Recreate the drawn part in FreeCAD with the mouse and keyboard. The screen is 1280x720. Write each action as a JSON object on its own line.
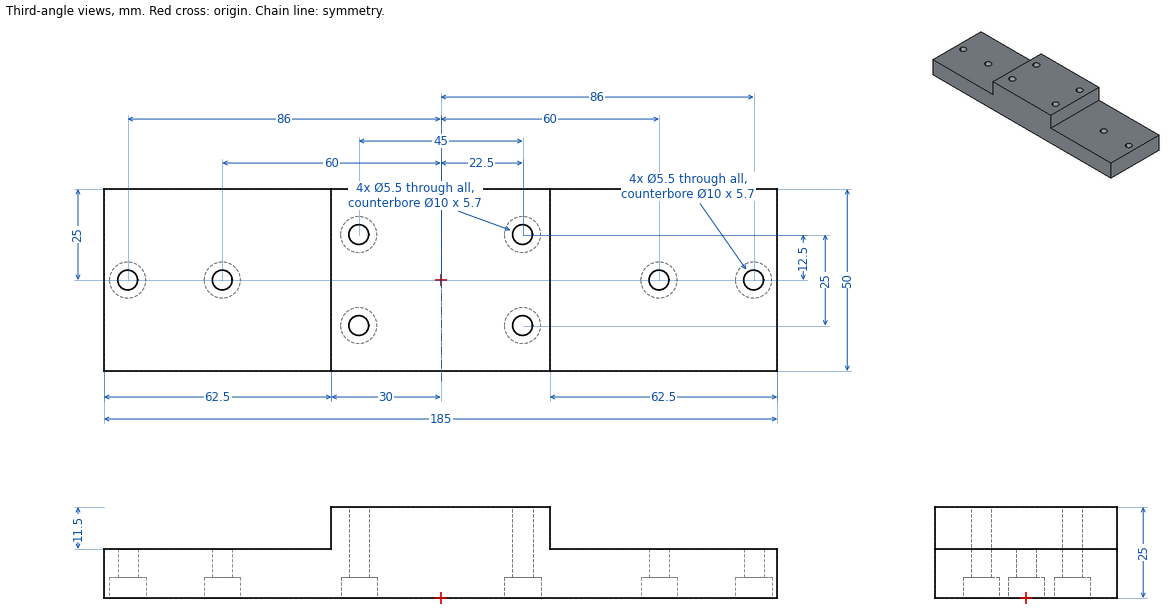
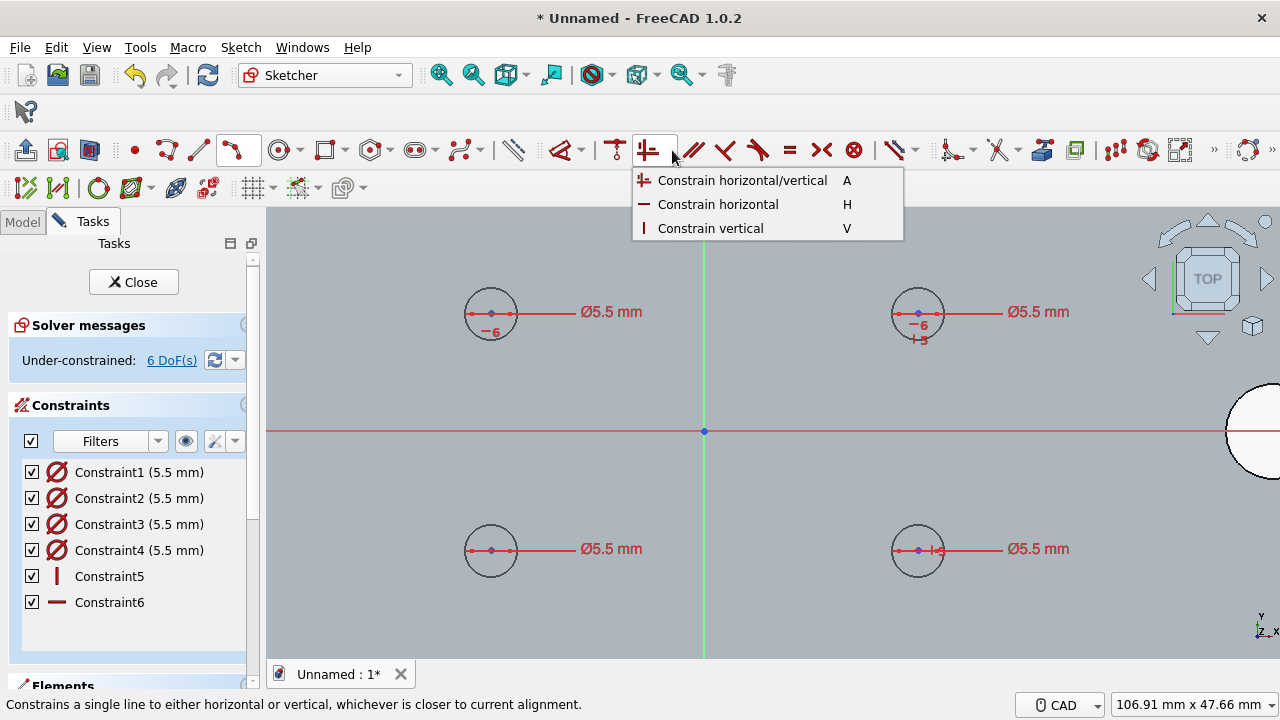
{"action": "left_click", "coordinate": [768, 228]}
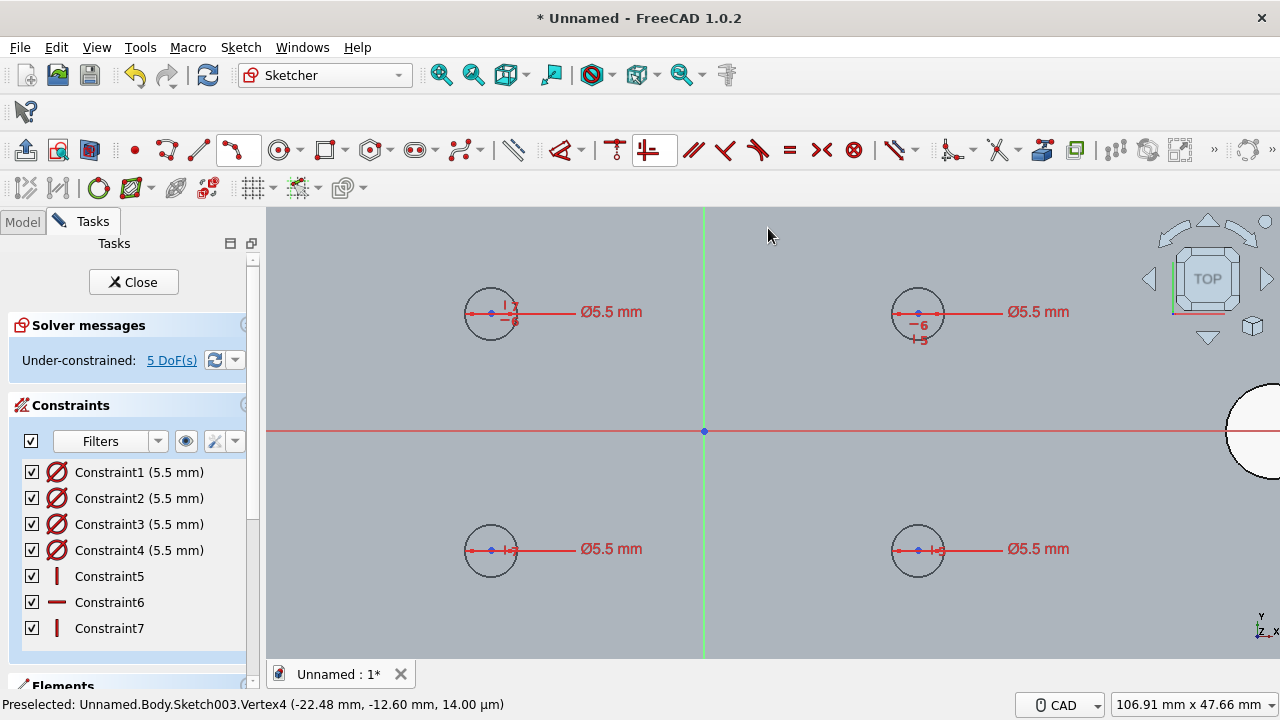
{"action": "left_click", "coordinate": [918, 551]}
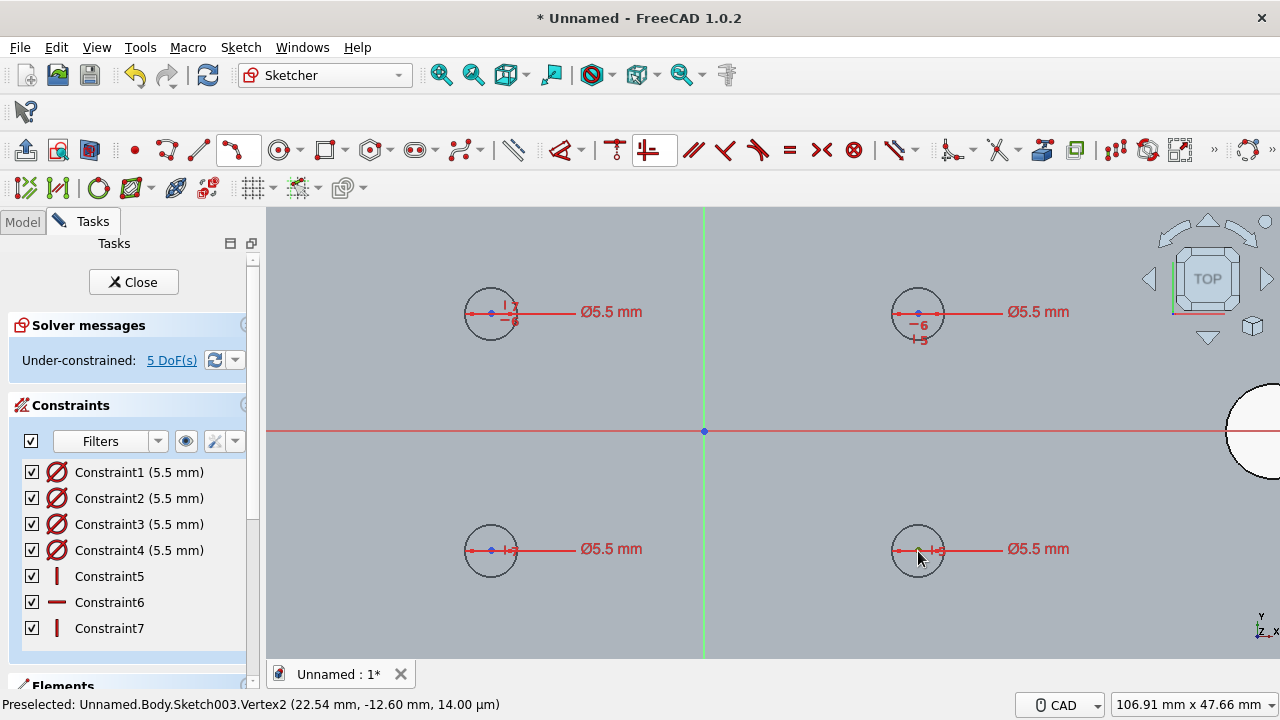
{"action": "left_click", "coordinate": [491, 551]}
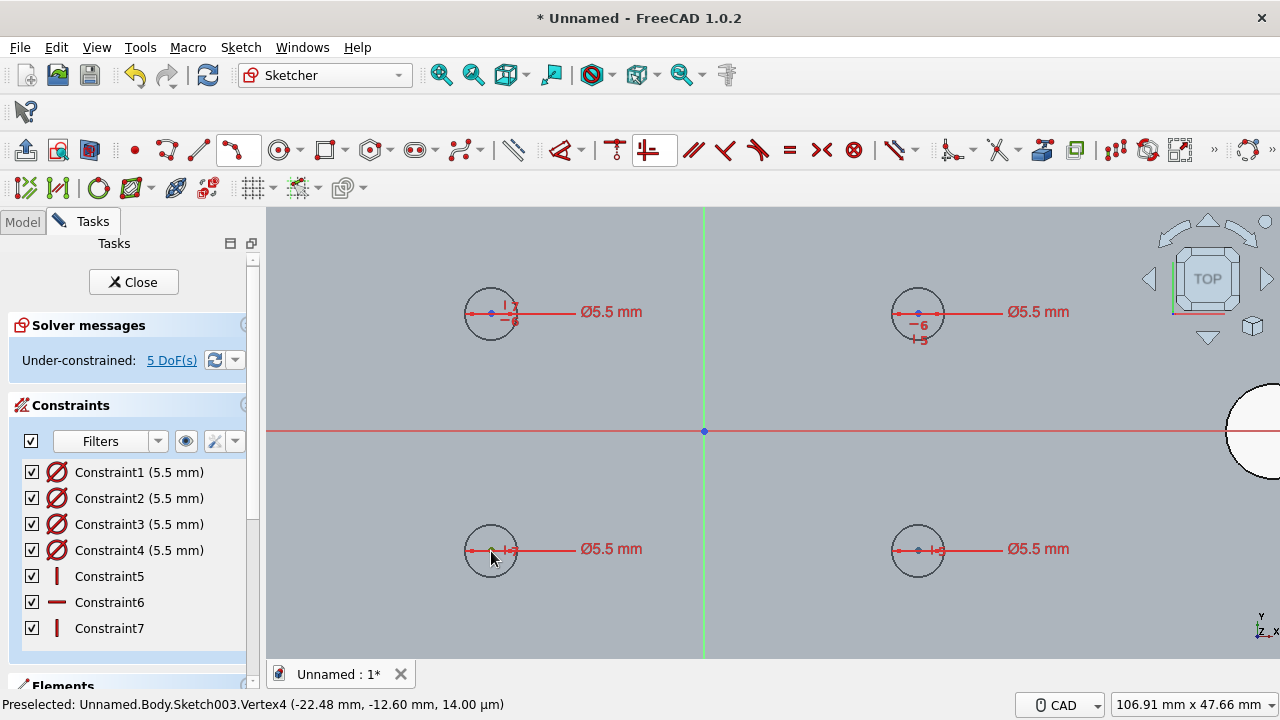
{"action": "left_click", "coordinate": [672, 150]}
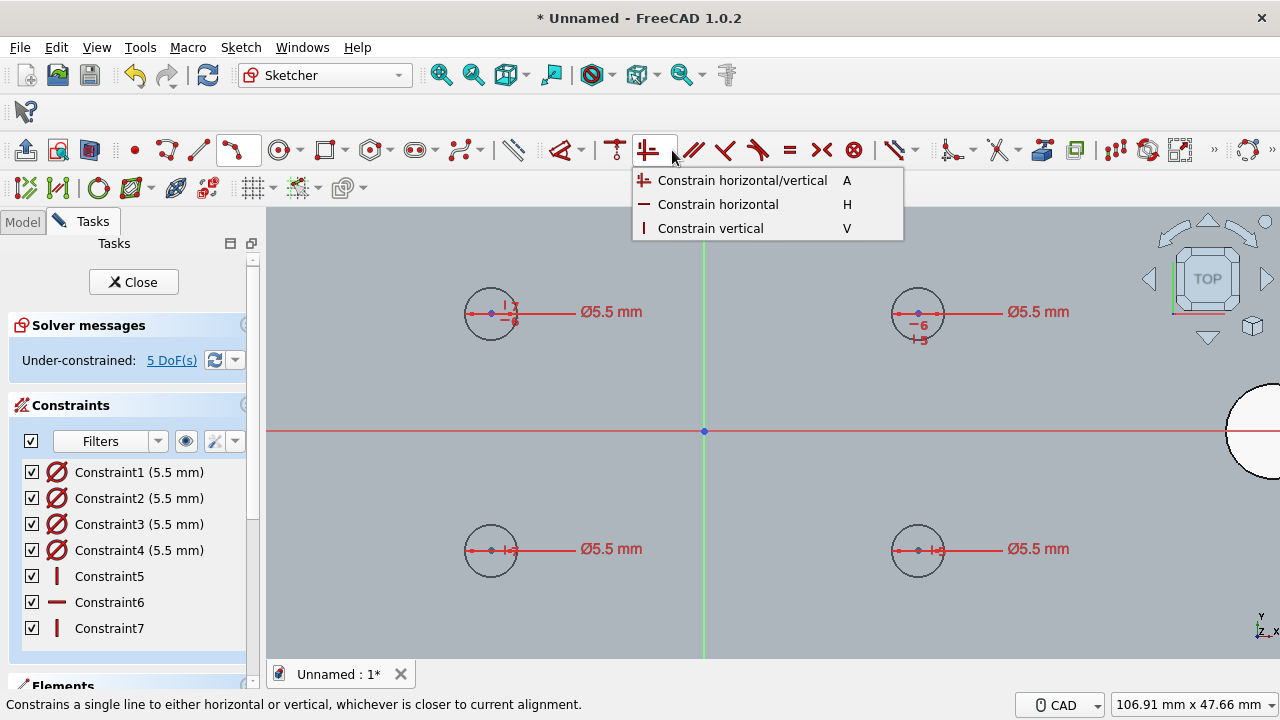
{"action": "left_click", "coordinate": [768, 204]}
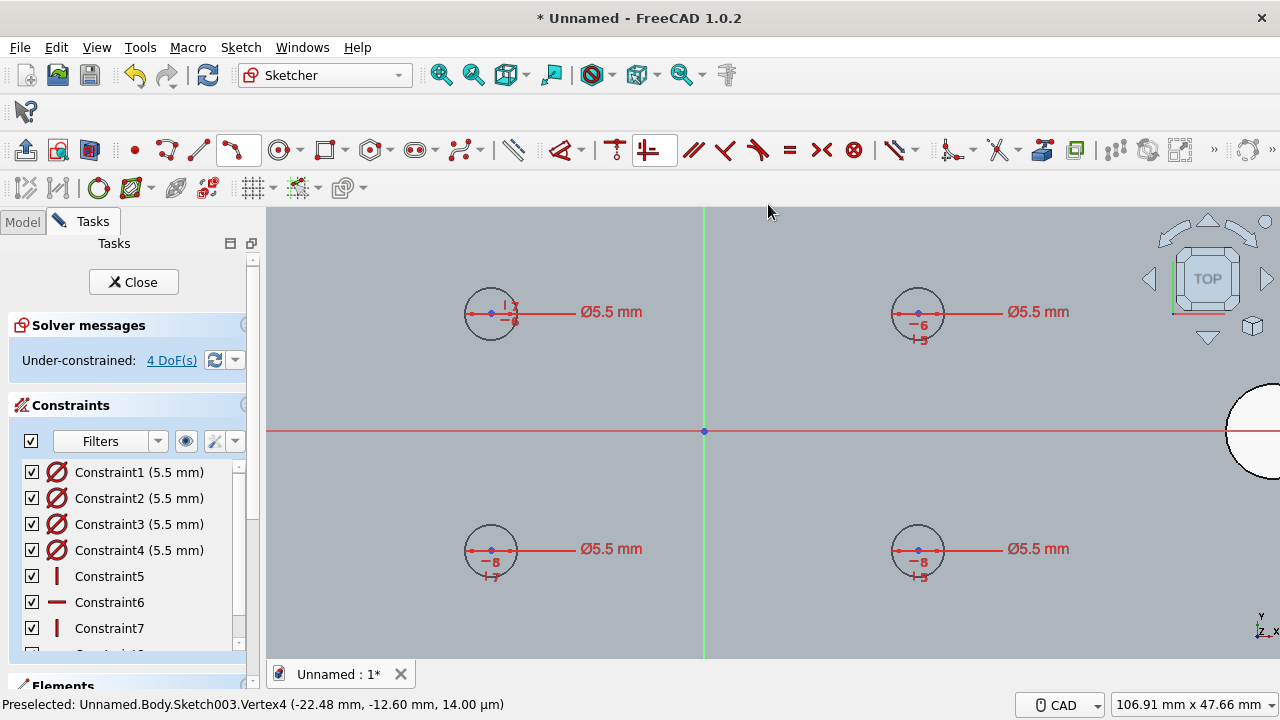
{"action": "left_click", "coordinate": [560, 150]}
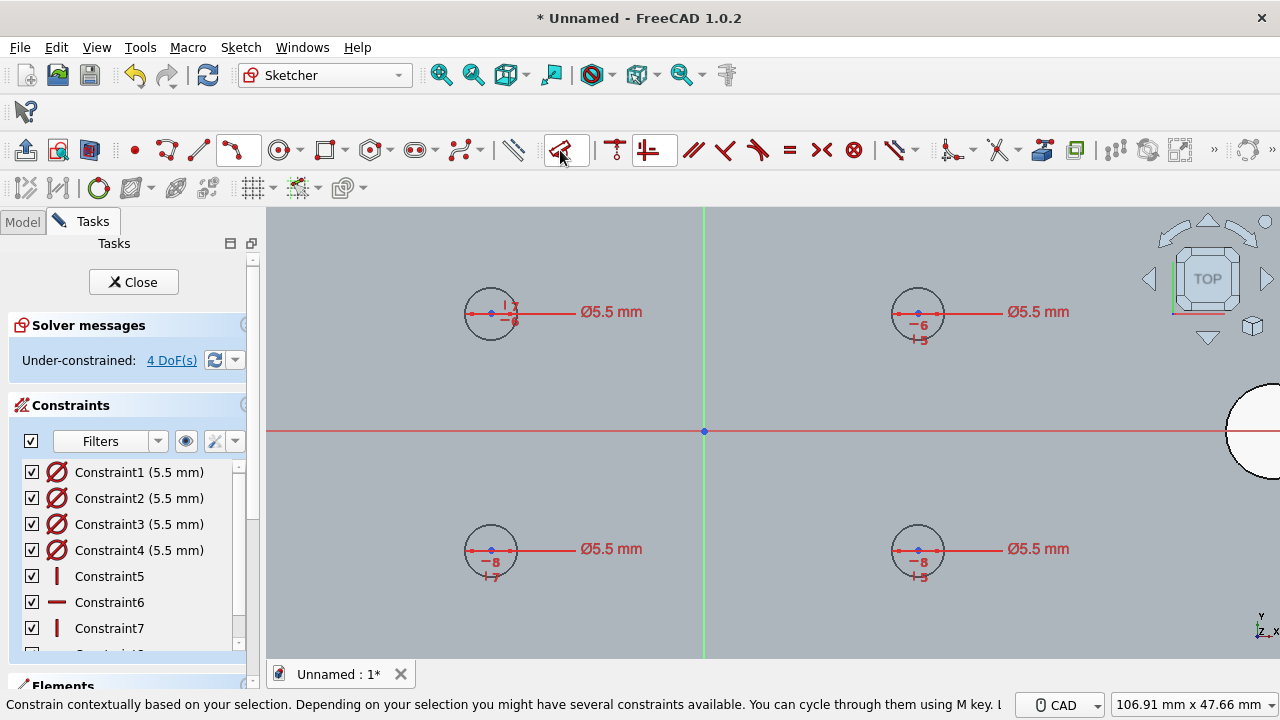
{"action": "left_click", "coordinate": [918, 314]}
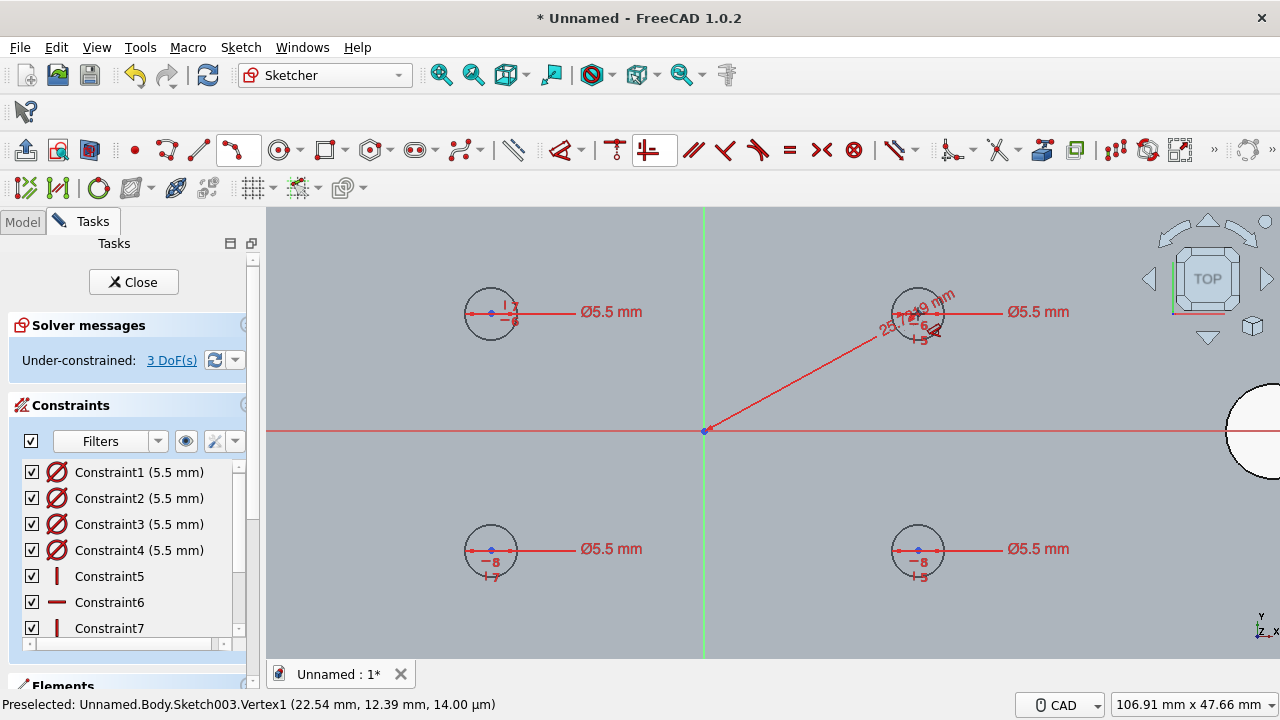
{"action": "left_click", "coordinate": [918, 551]}
{"action": "left_click", "coordinate": [952, 378]}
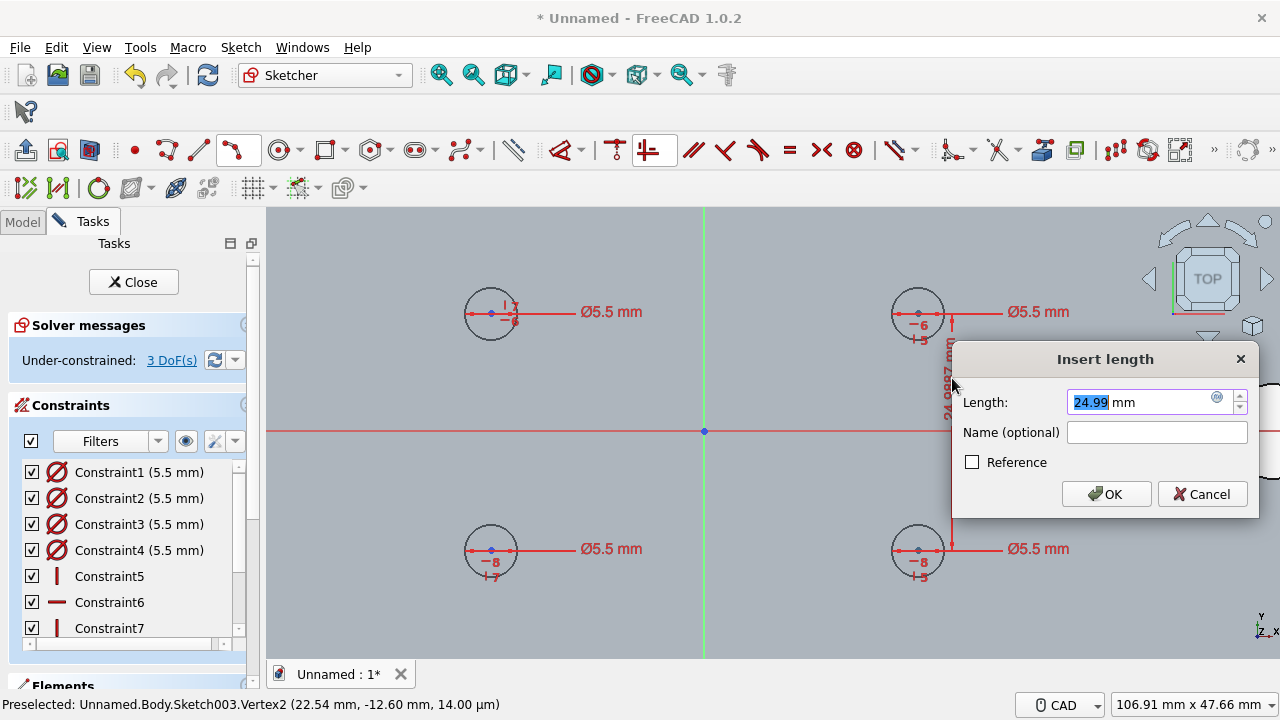
{"action": "type", "text": "25"}
{"action": "key", "text": "Return"}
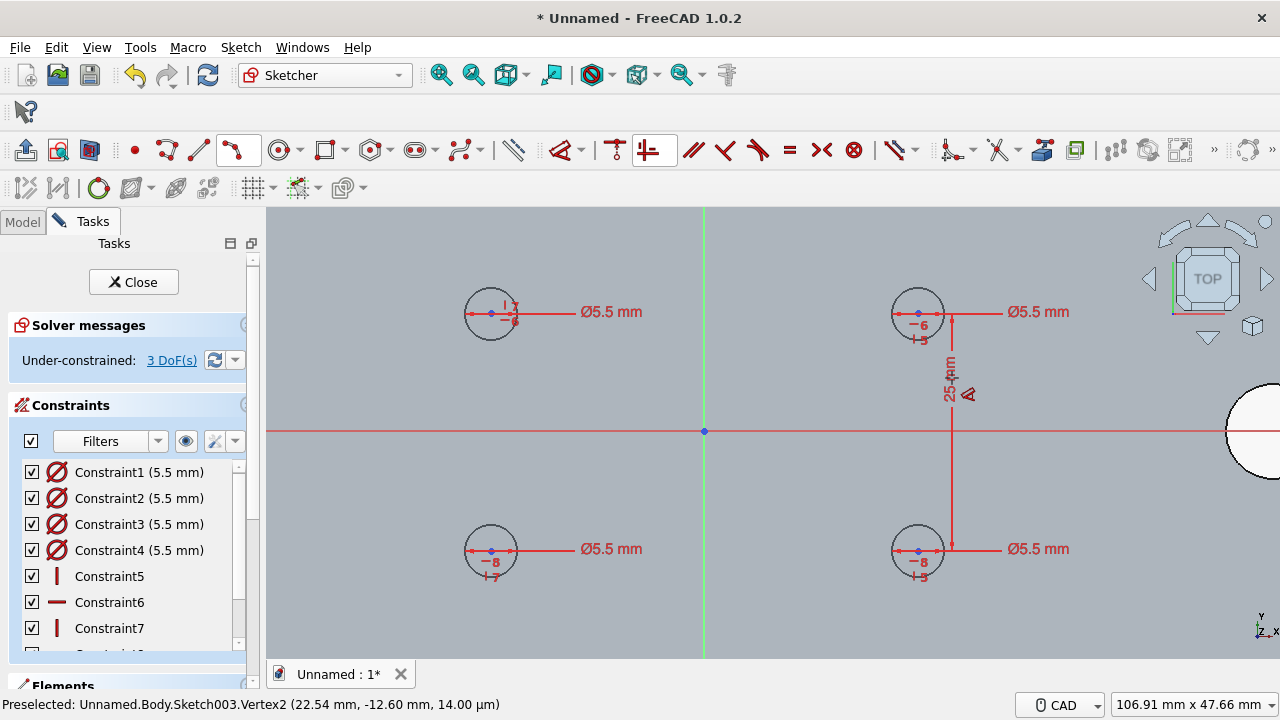
{"action": "left_click", "coordinate": [918, 314]}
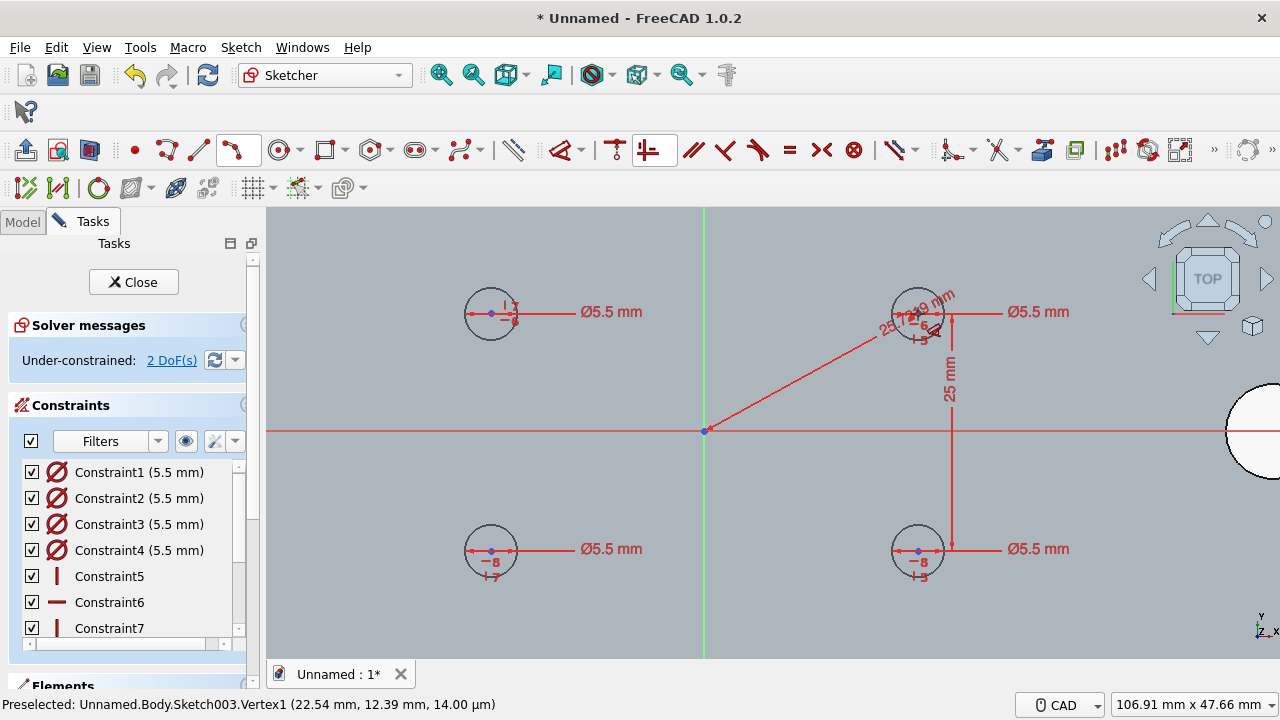
{"action": "left_click", "coordinate": [491, 314]}
{"action": "left_click", "coordinate": [606, 280]}